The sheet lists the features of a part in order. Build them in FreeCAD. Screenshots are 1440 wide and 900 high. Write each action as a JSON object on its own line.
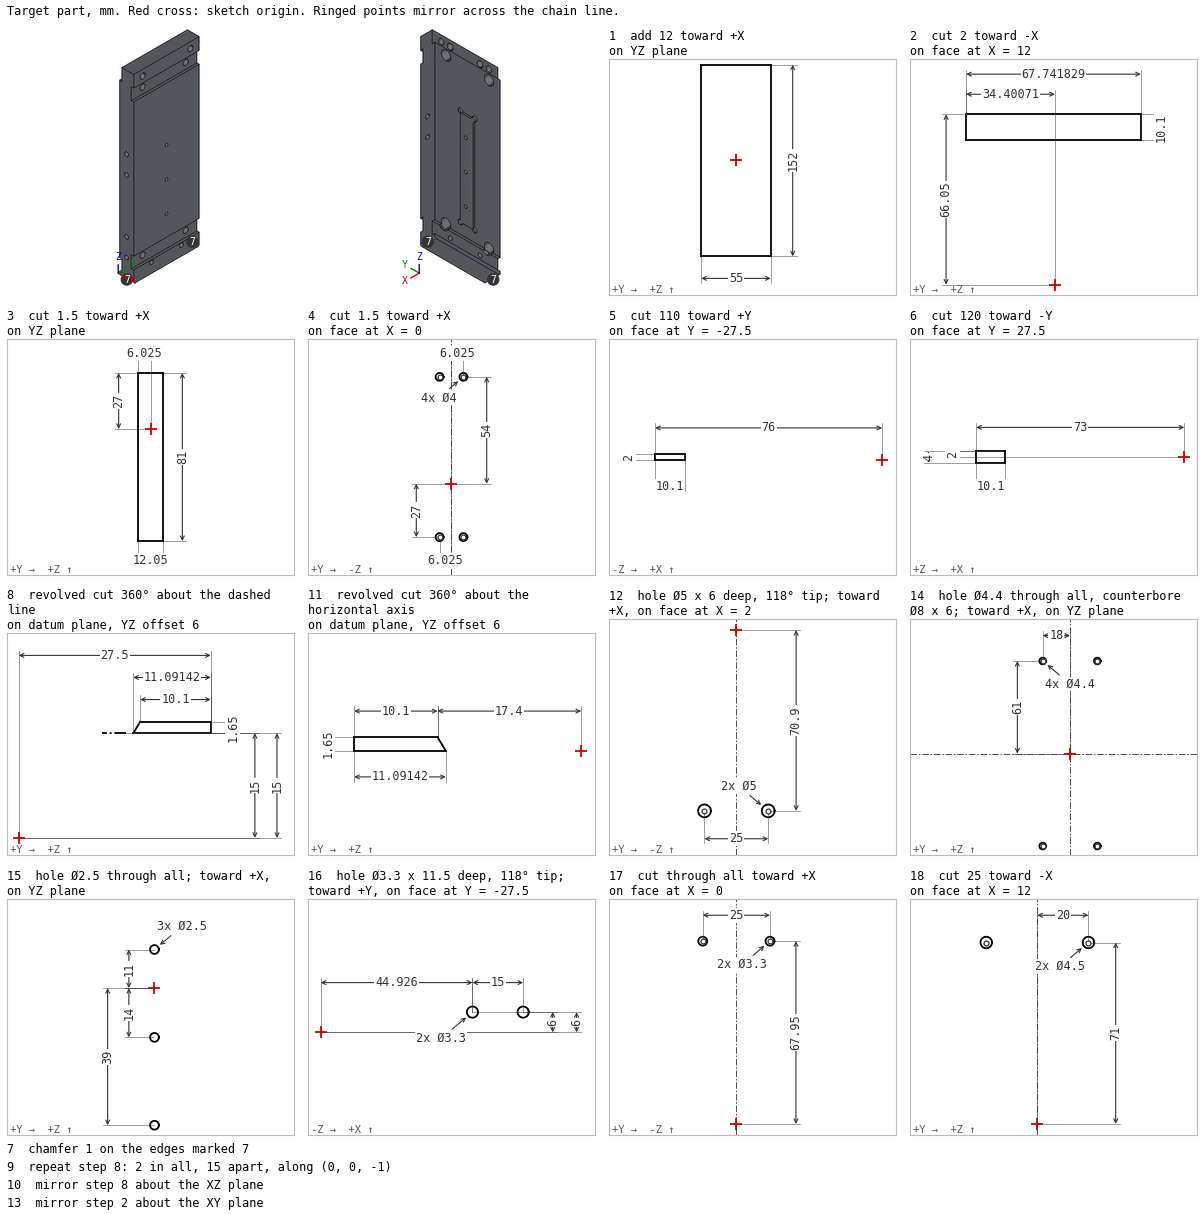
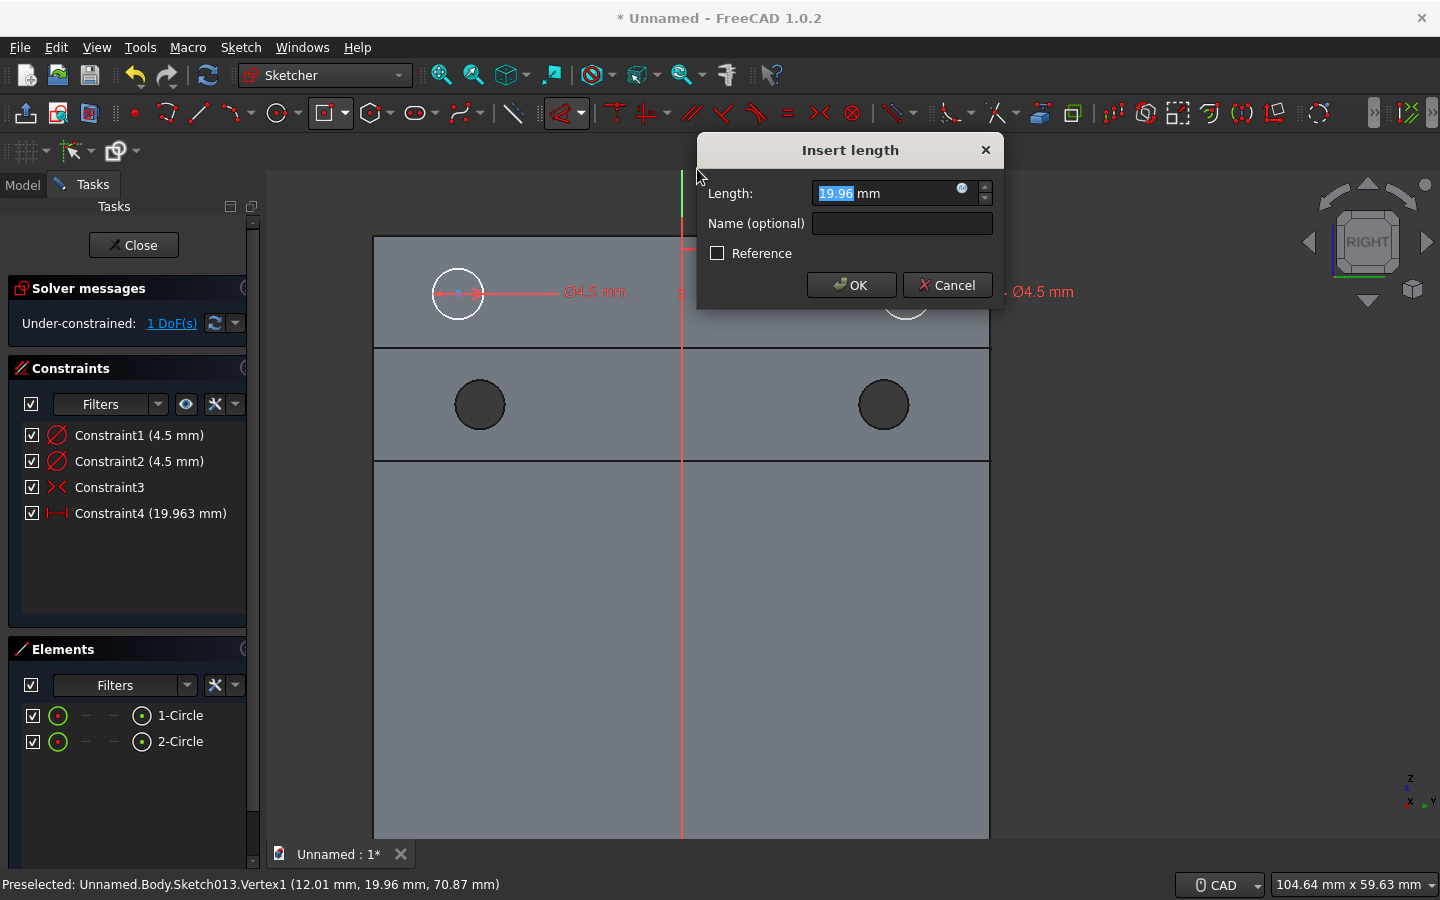
{"action": "type", "text": "20"}
{"action": "key", "text": "Return"}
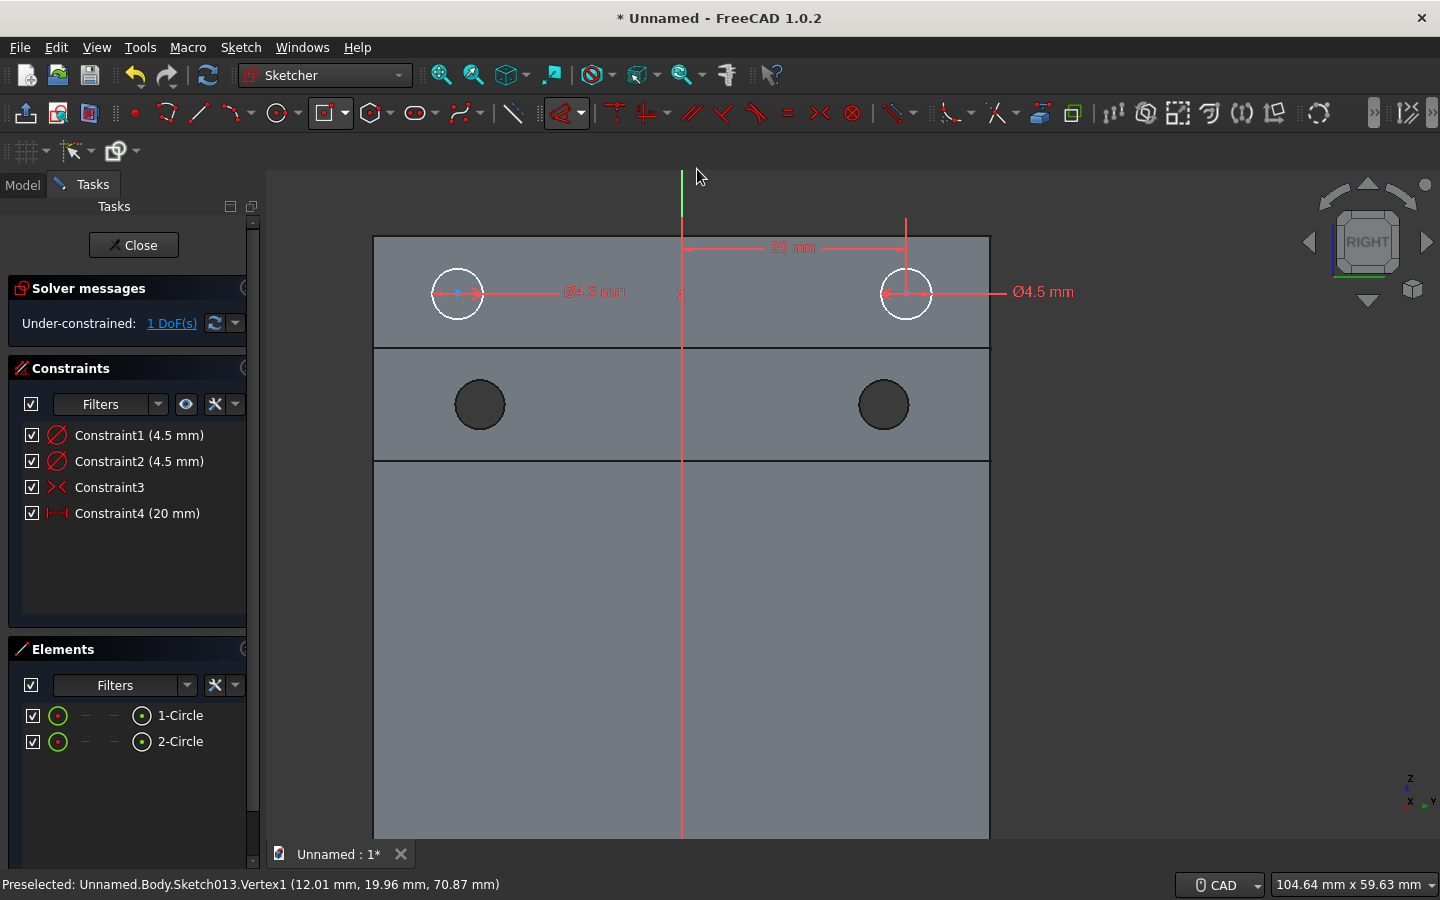
{"action": "left_click", "coordinate": [906, 294]}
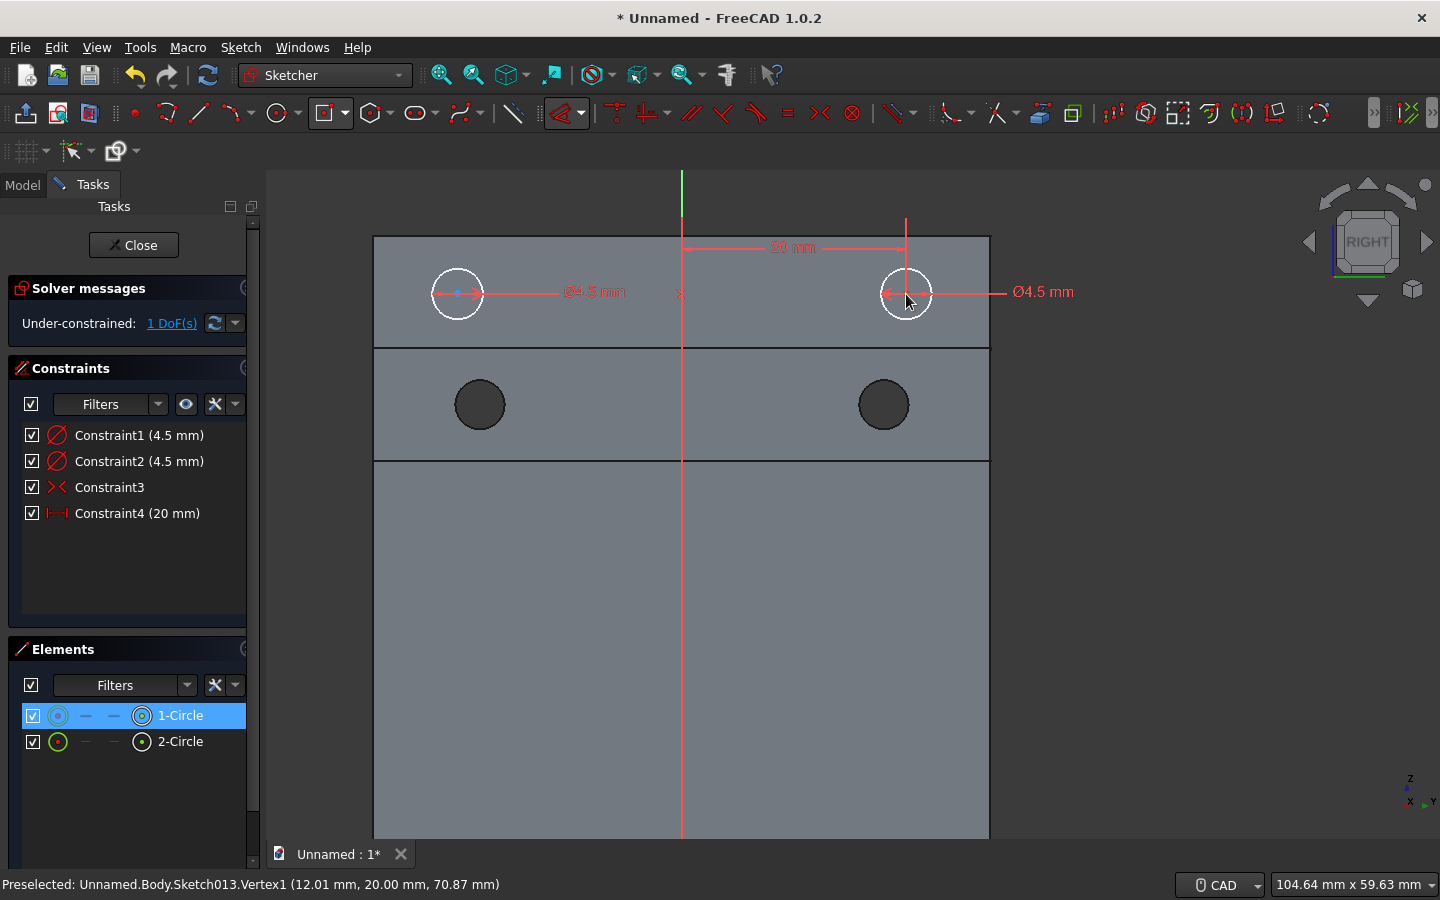
{"action": "key", "text": "i"}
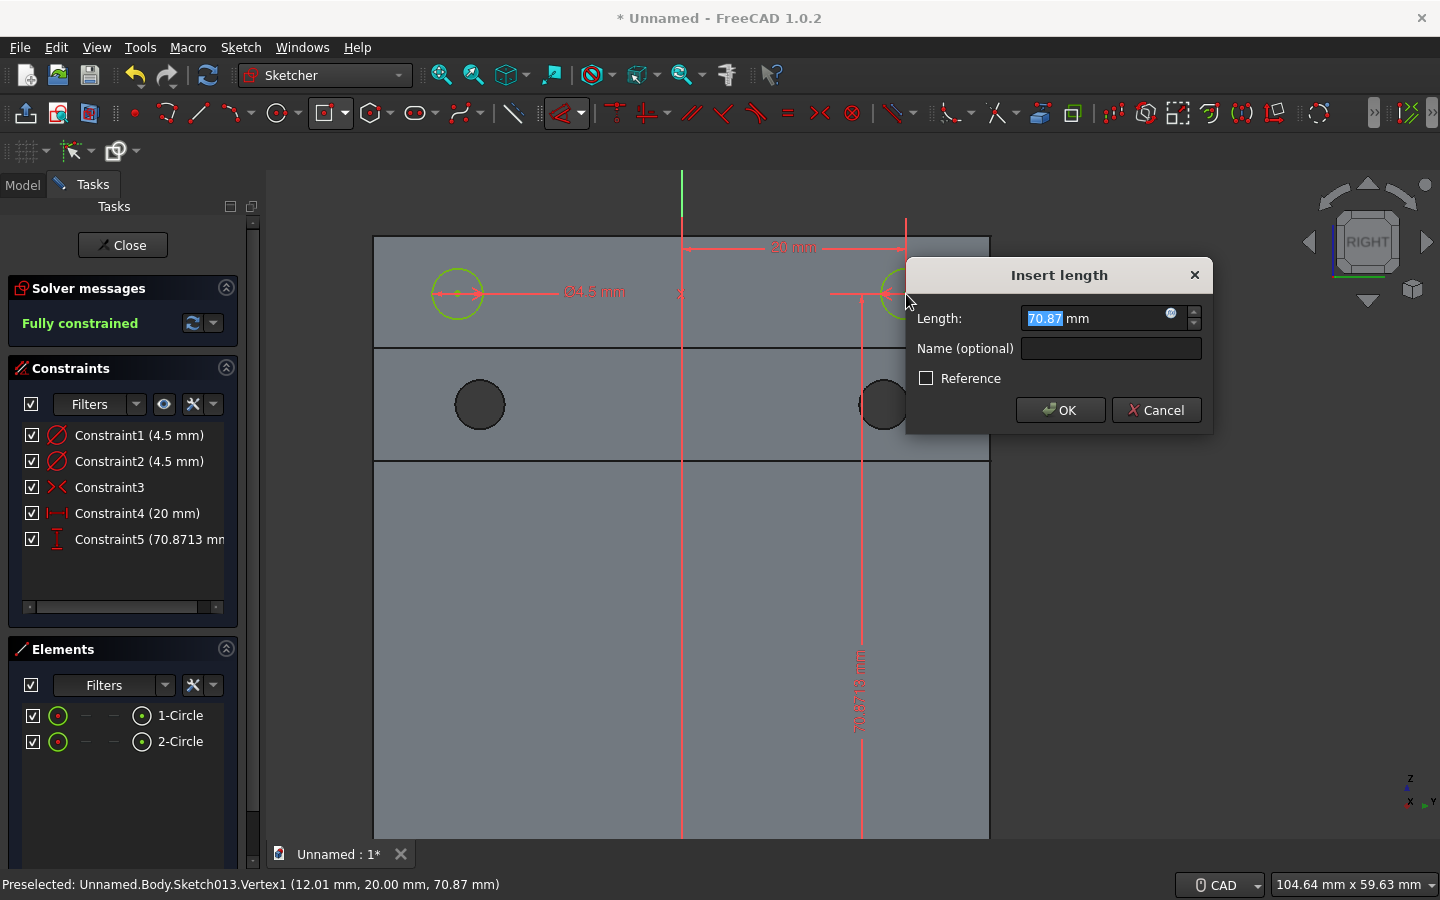
{"action": "type", "text": "71"}
{"action": "key", "text": "Return"}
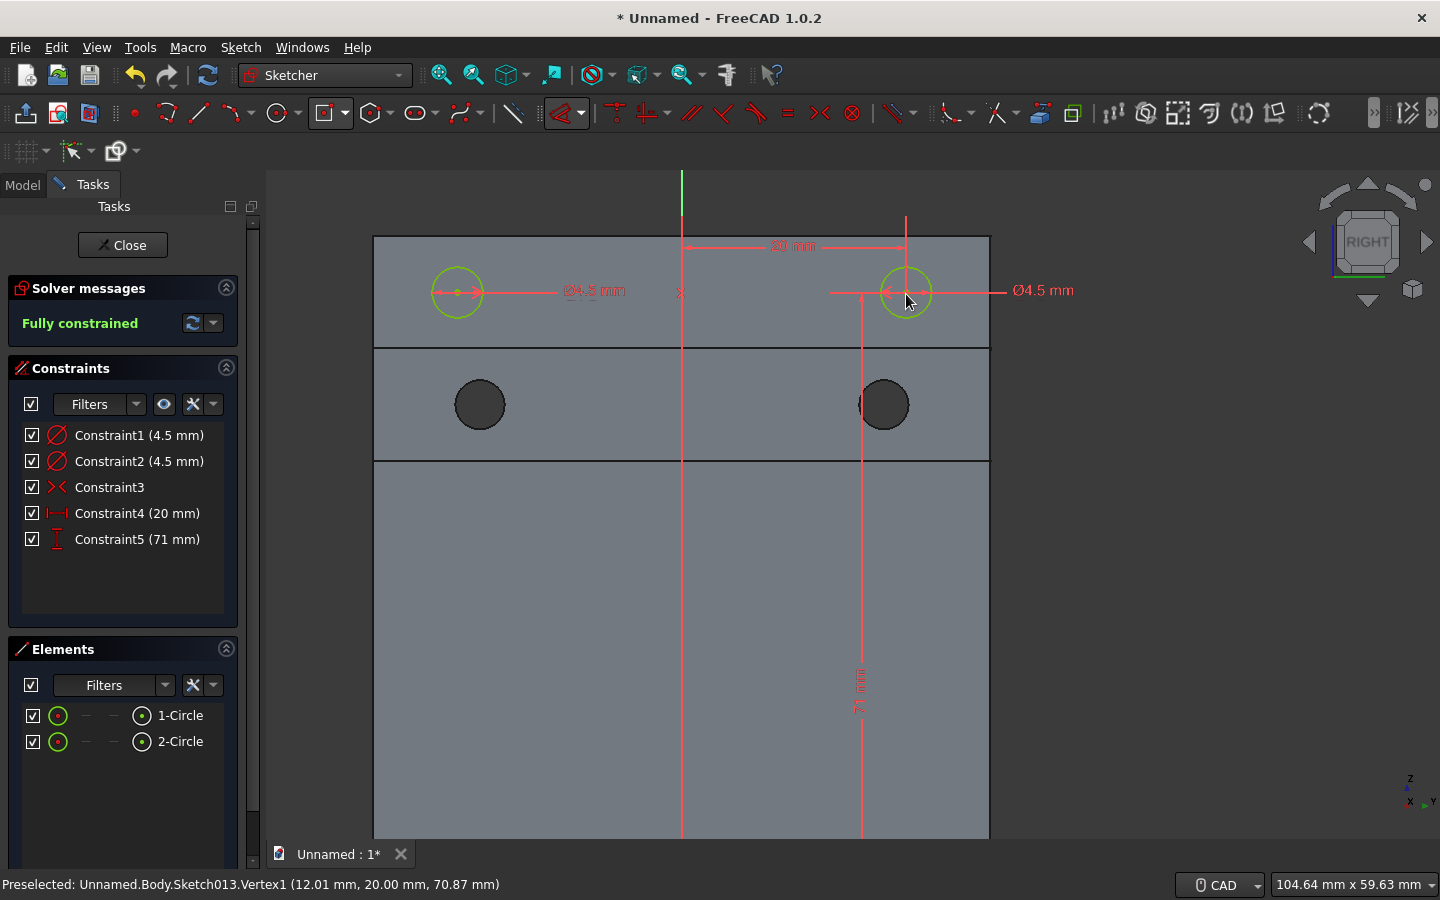
{"action": "left_click", "coordinate": [123, 245]}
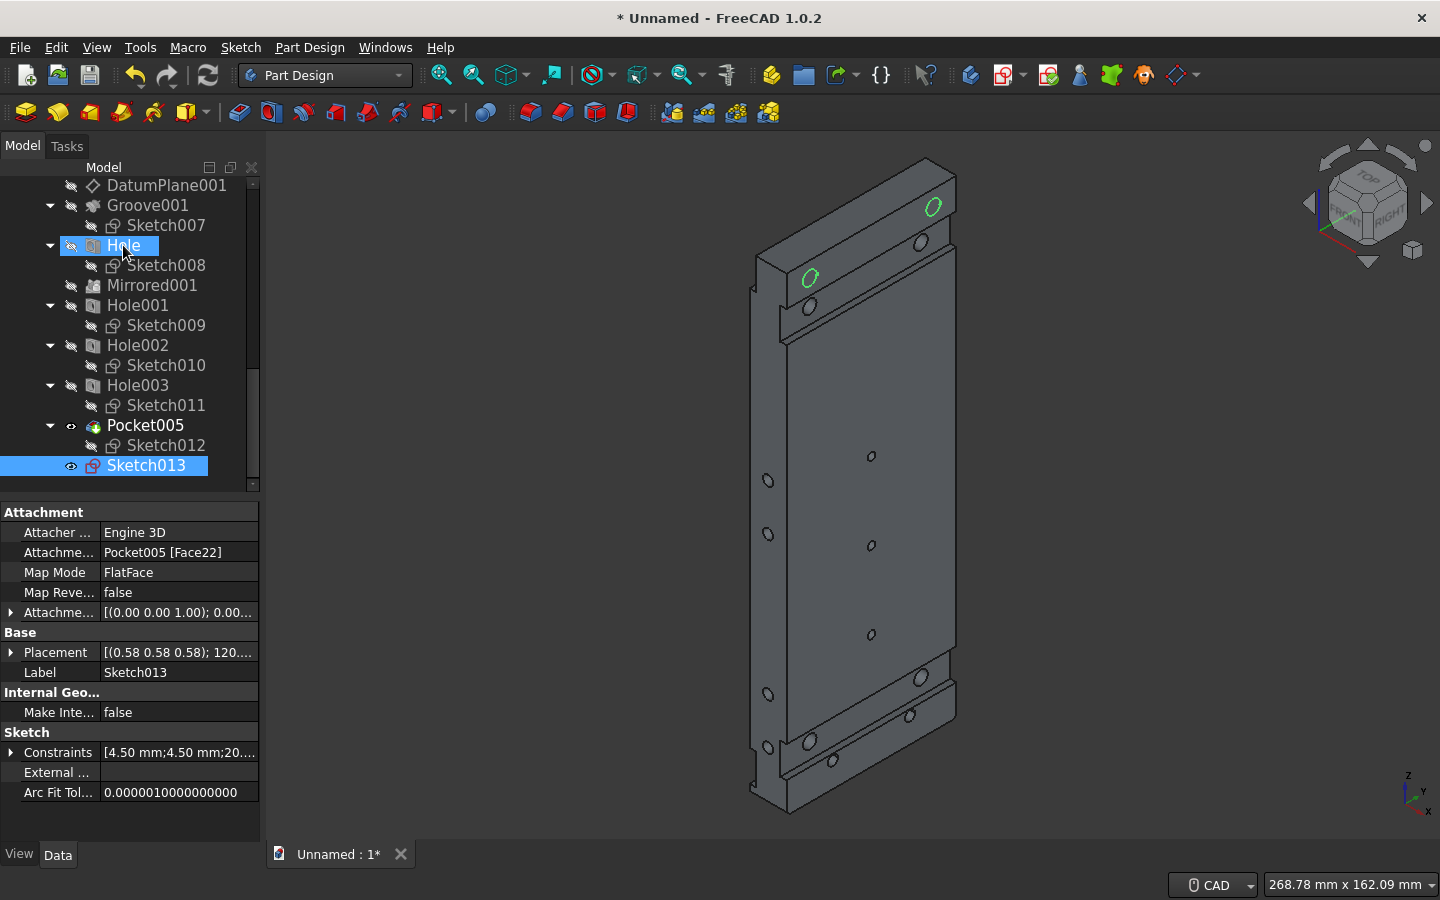
{"action": "left_click", "coordinate": [240, 112]}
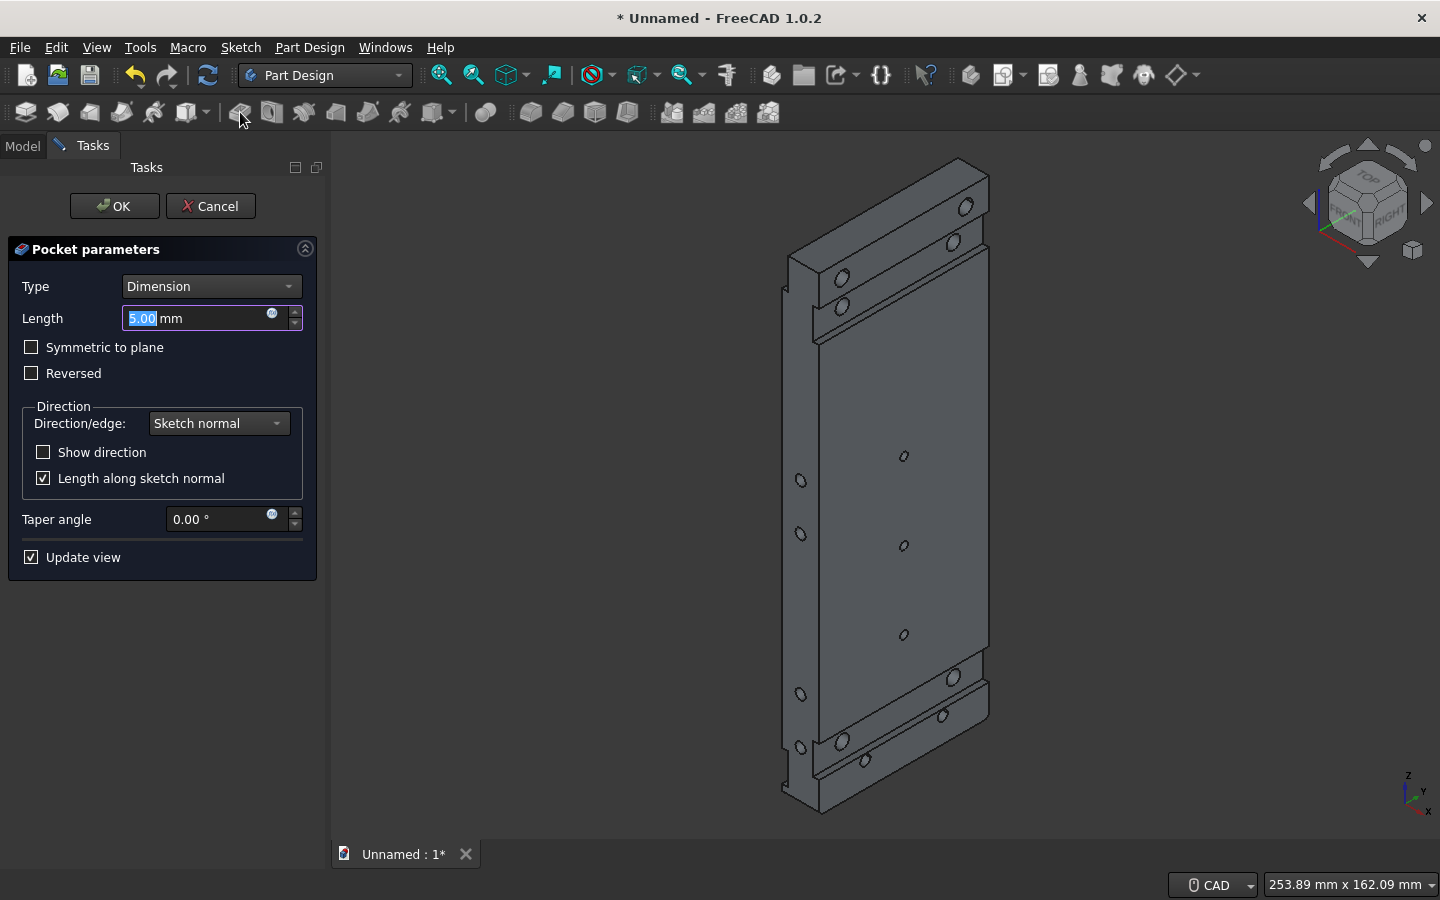
{"action": "type", "text": "25"}
{"action": "key", "text": "Tab"}